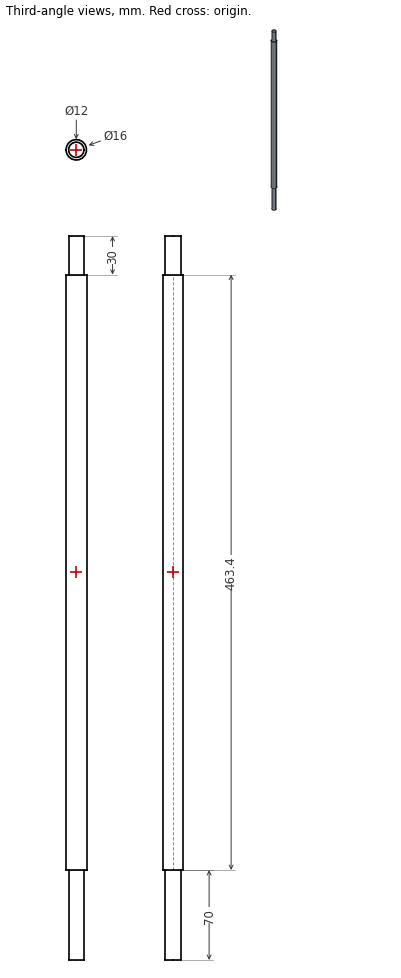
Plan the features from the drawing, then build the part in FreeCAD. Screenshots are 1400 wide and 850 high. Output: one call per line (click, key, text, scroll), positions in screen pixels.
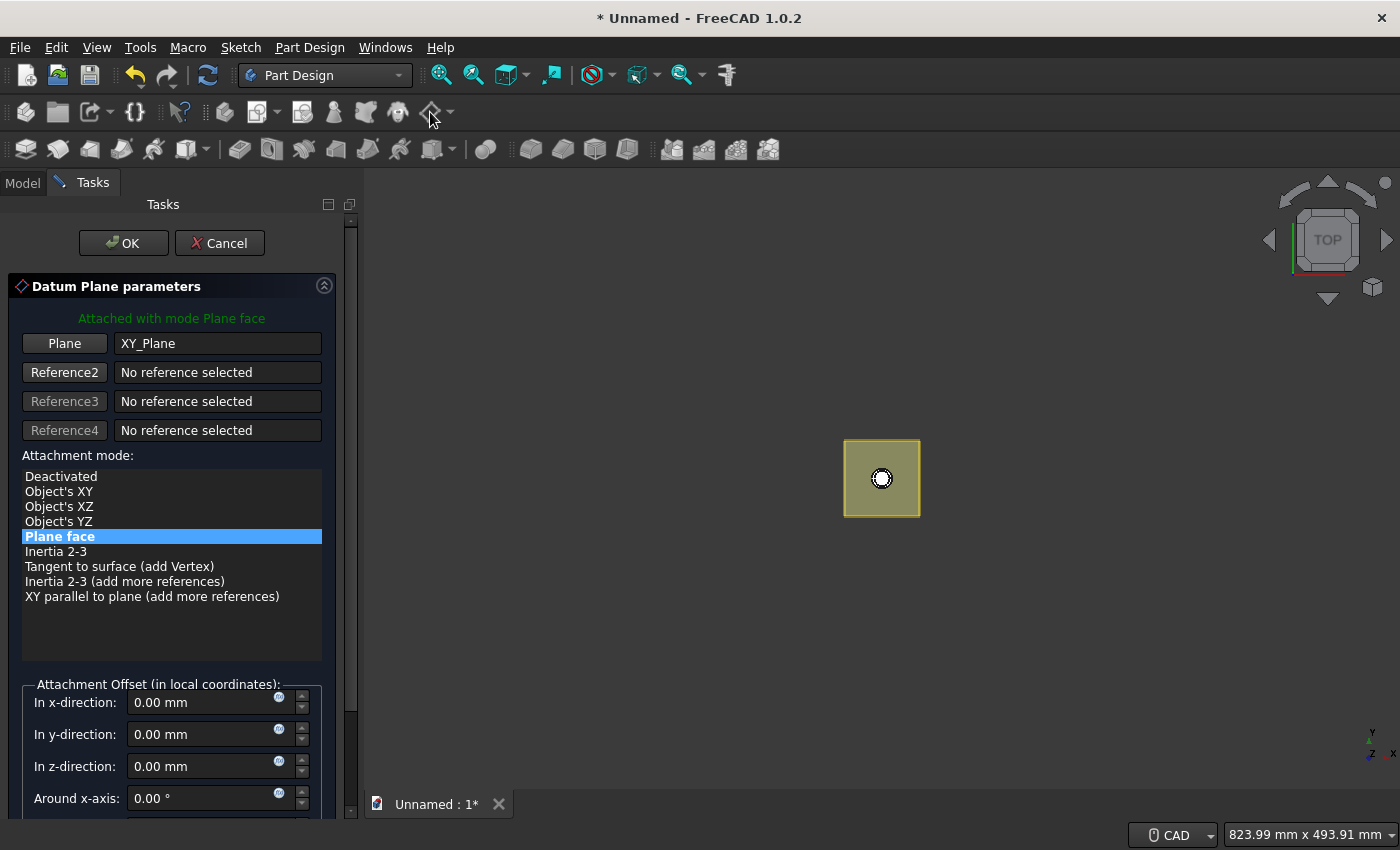
triple_click(210, 766)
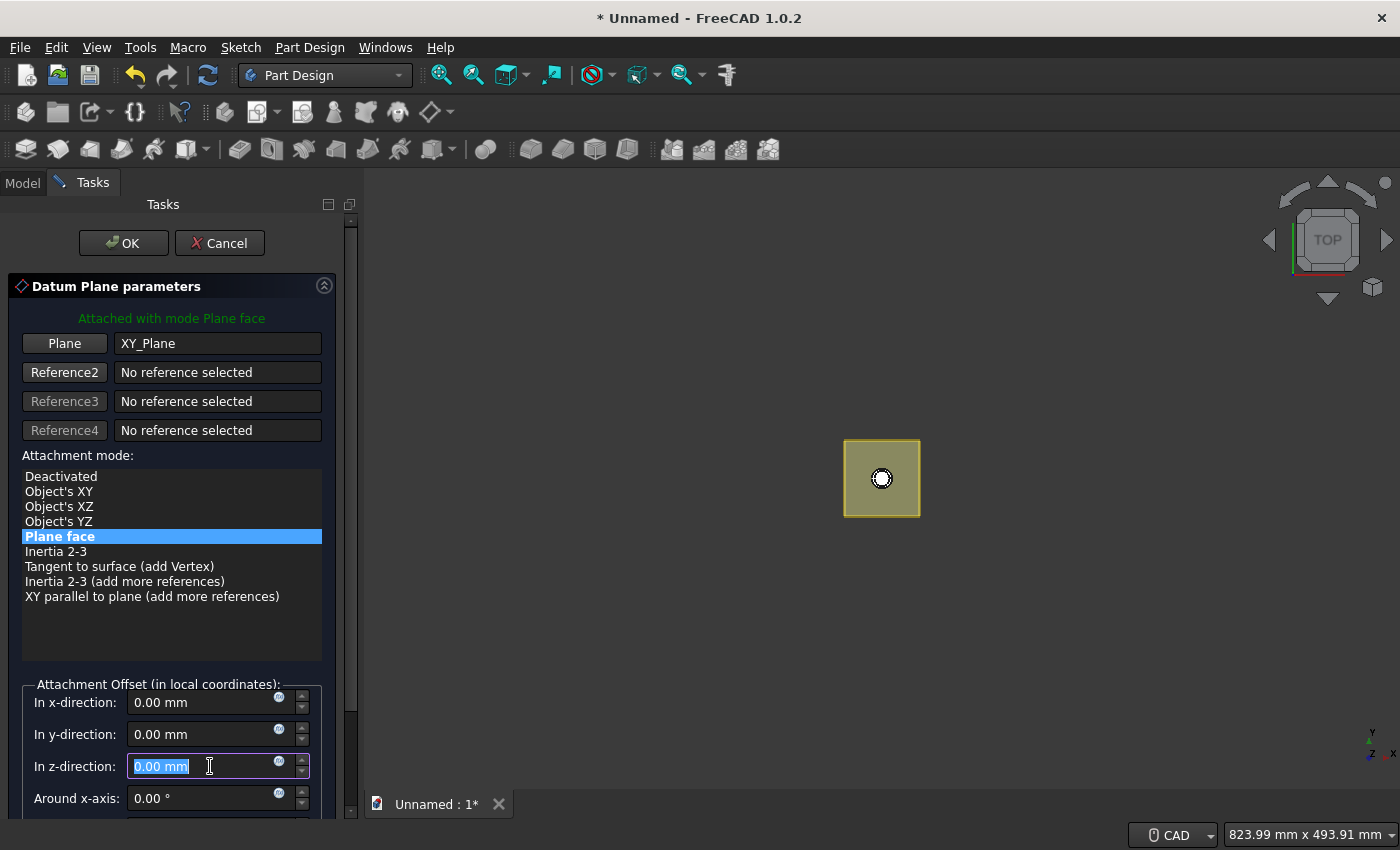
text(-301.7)
key(Tab)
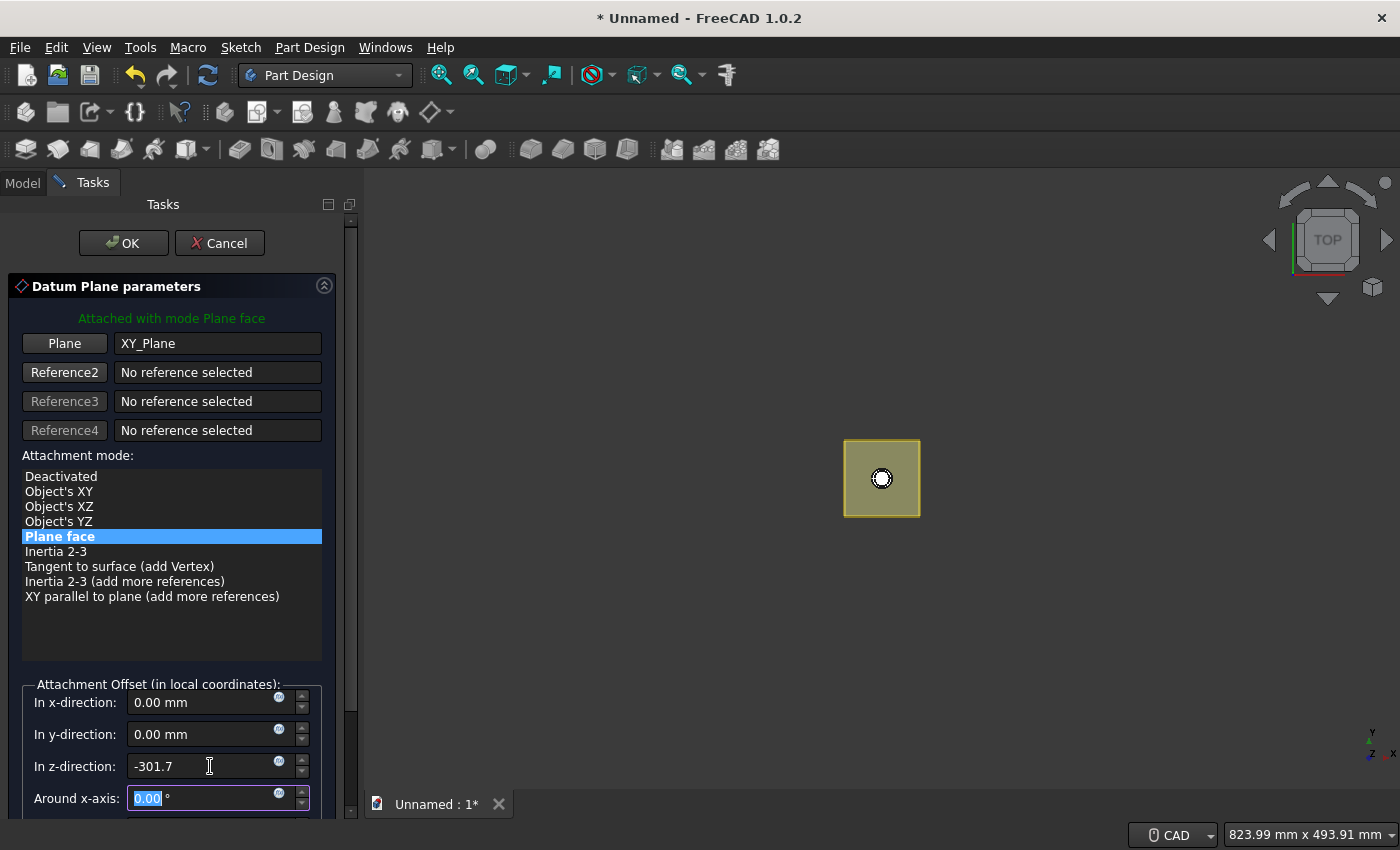
click(124, 243)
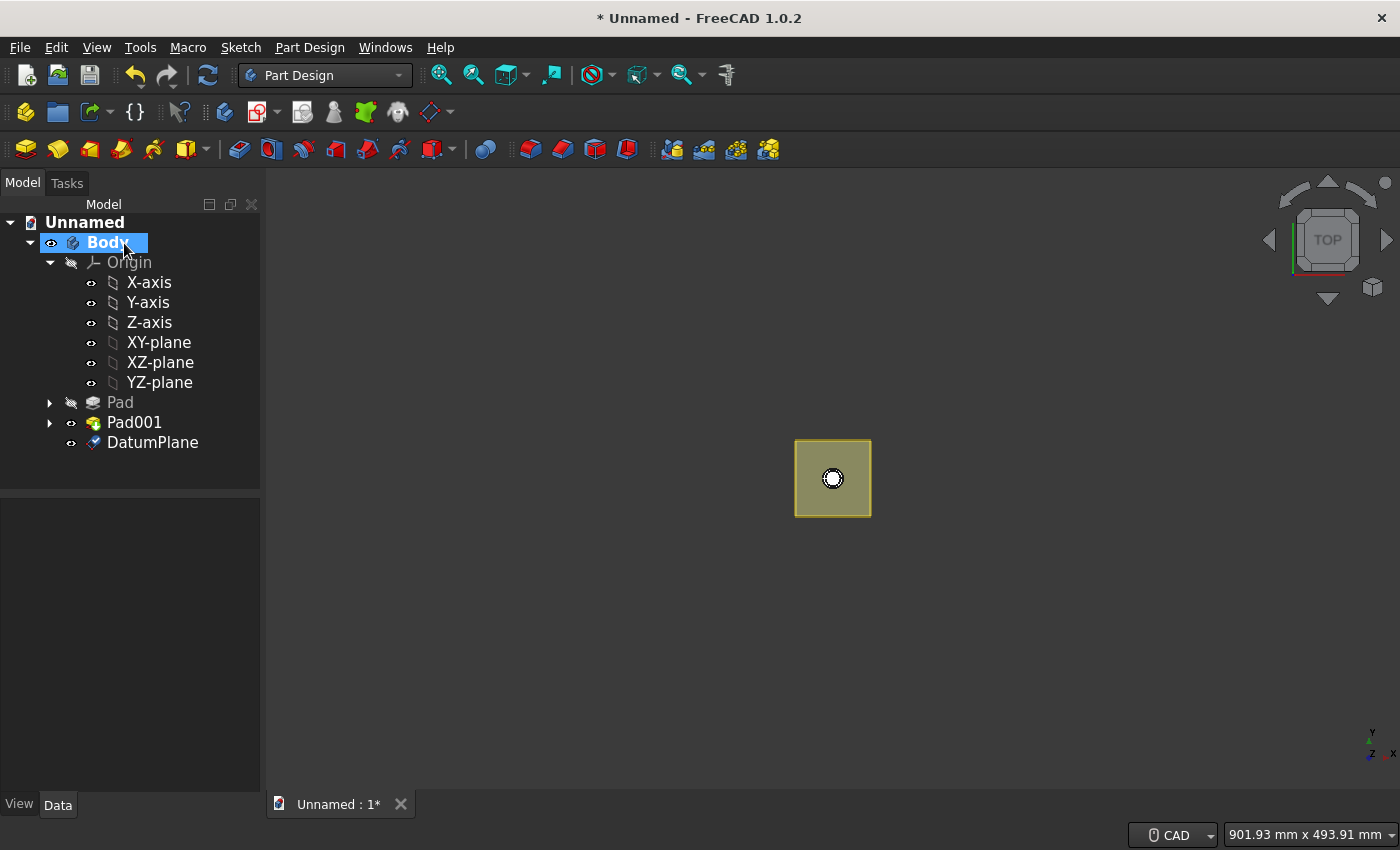
click(116, 443)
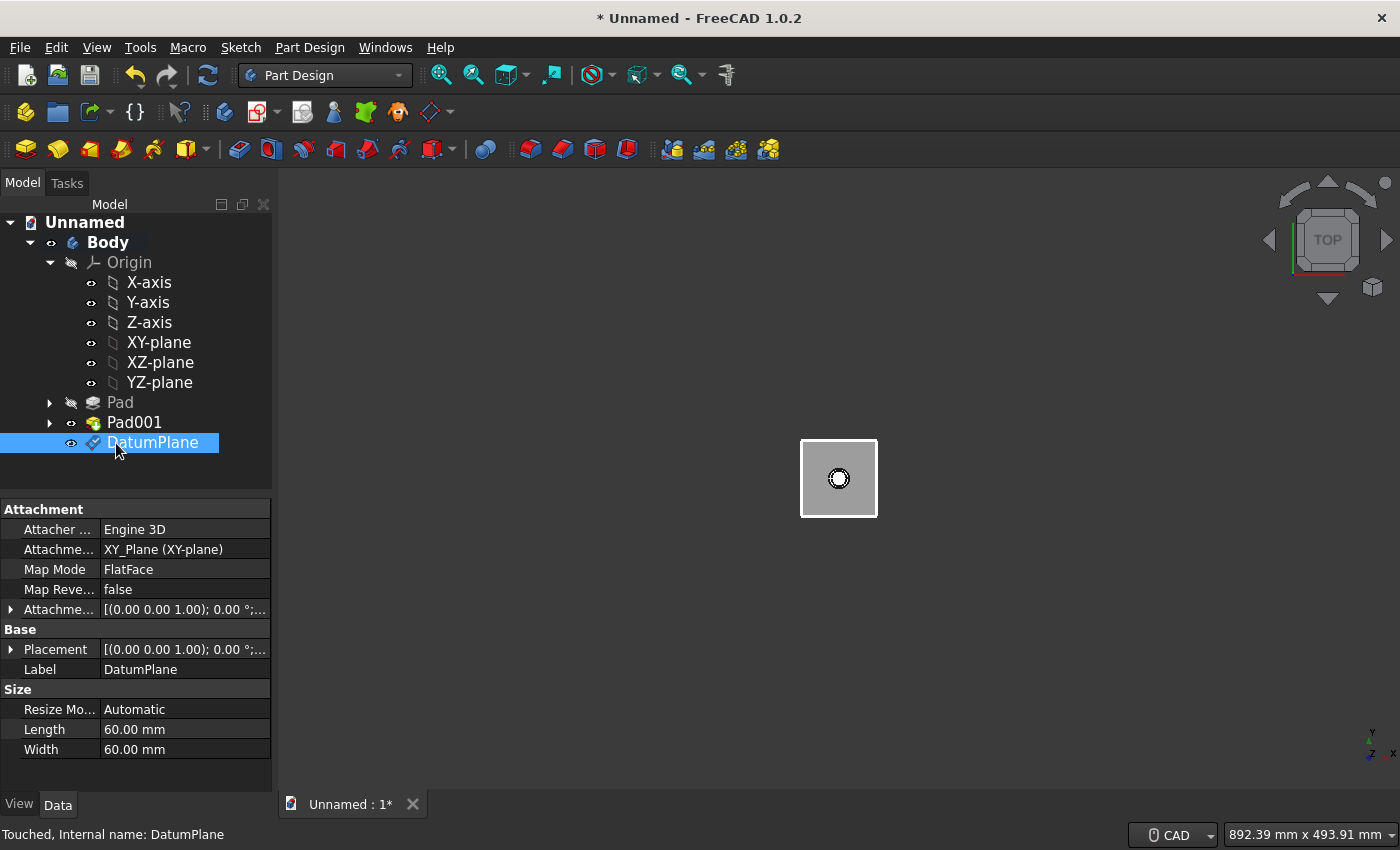
click(258, 112)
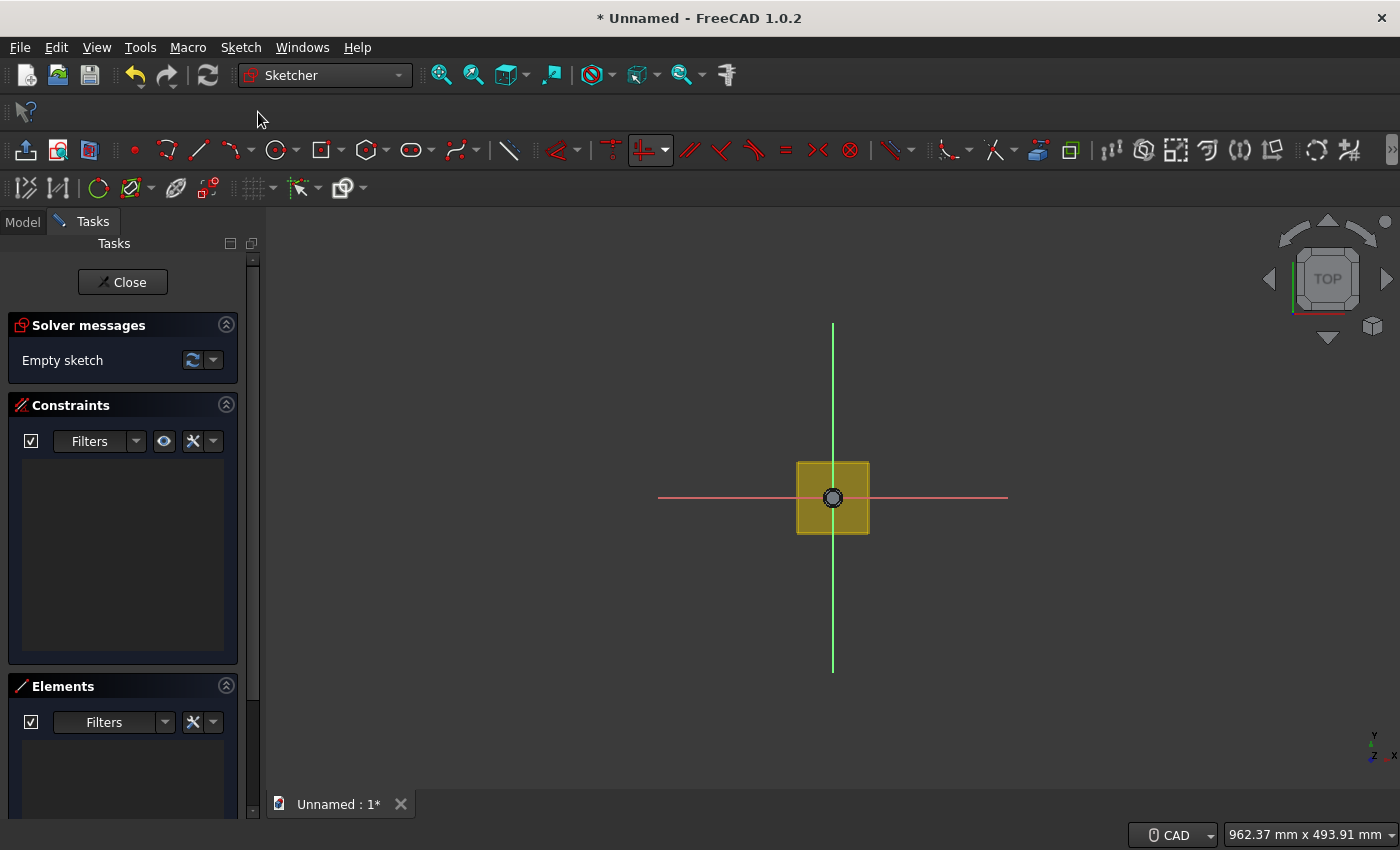
click(90, 150)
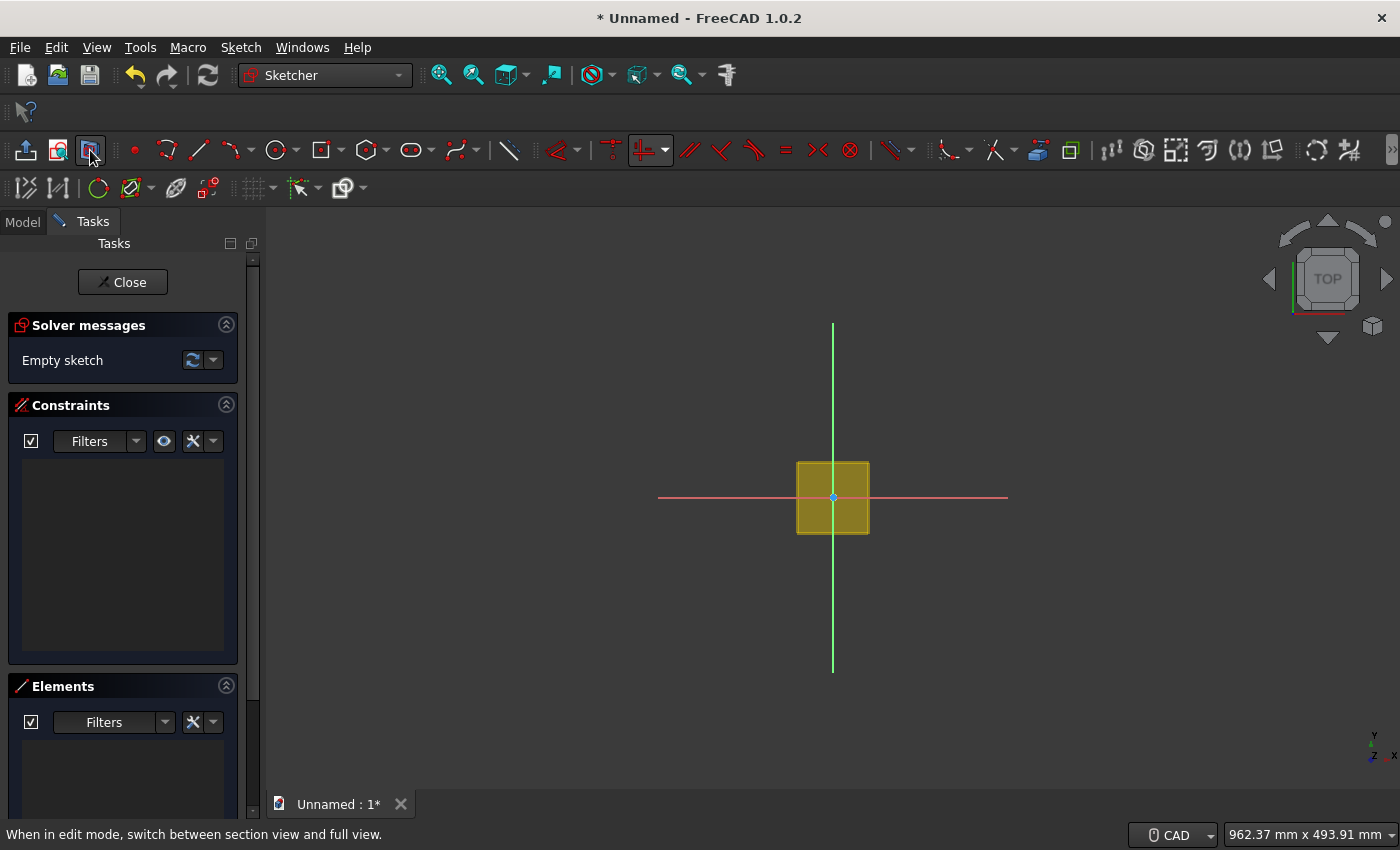
scroll(837, 498, up, 15)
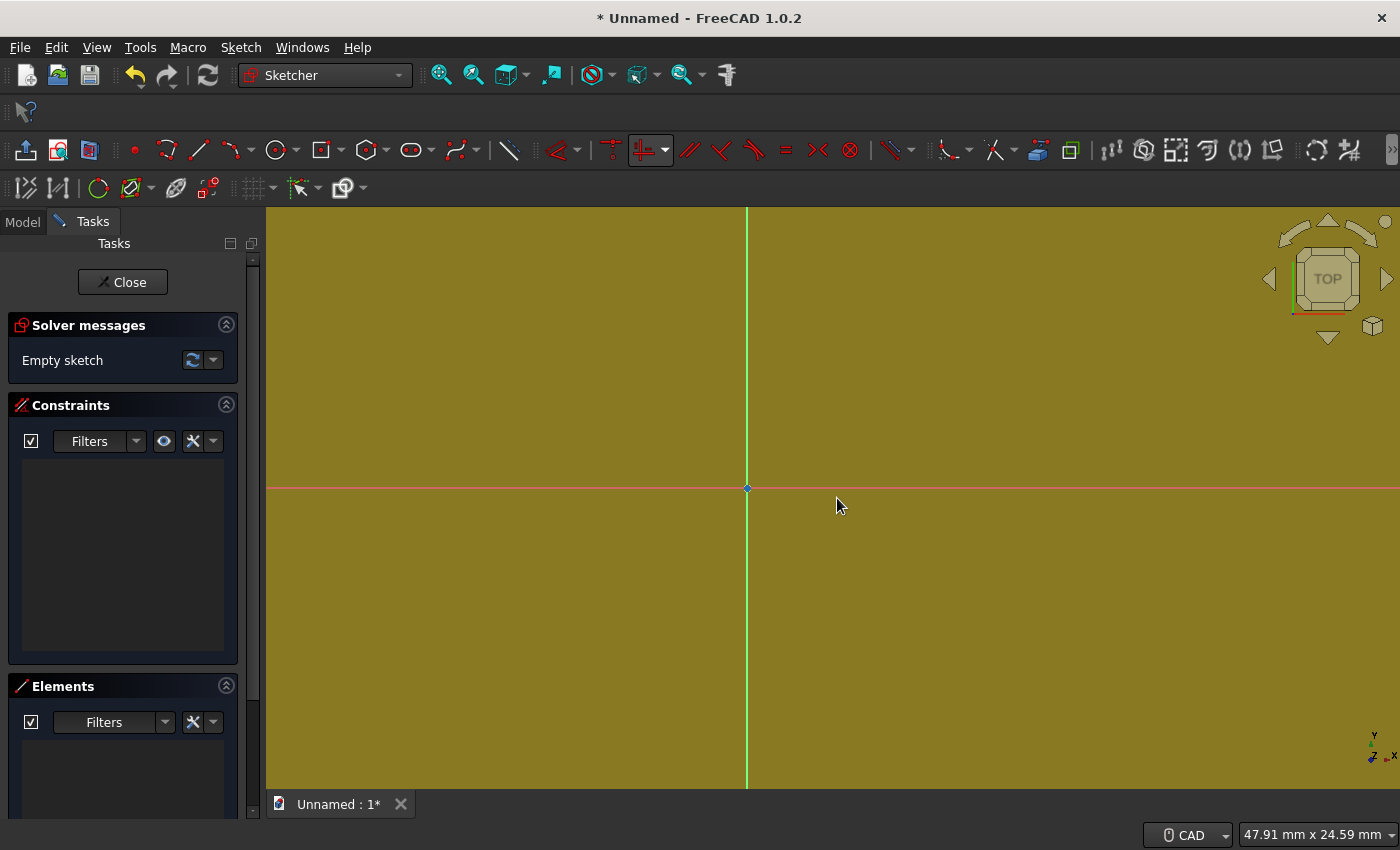
click(276, 150)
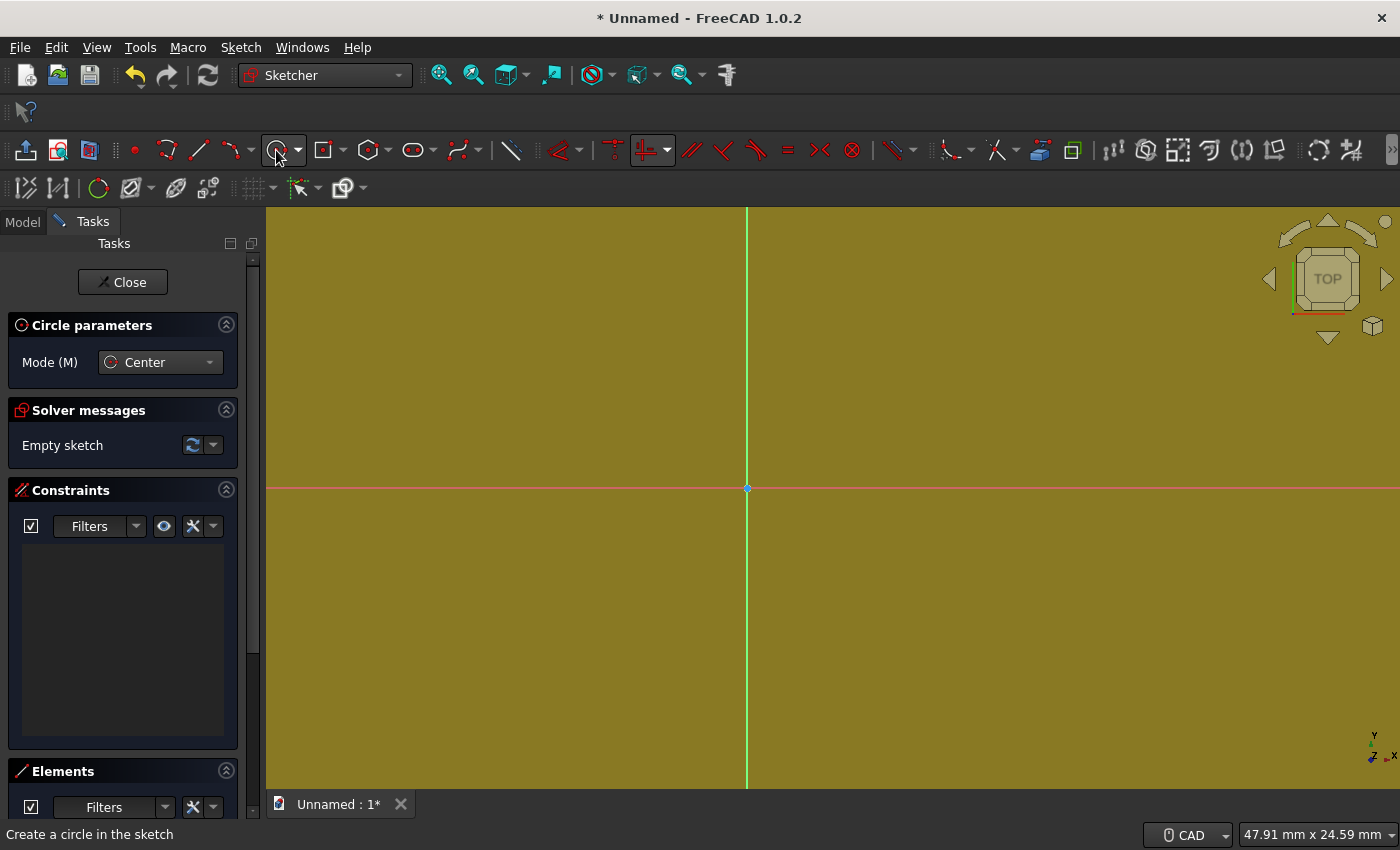
click(747, 488)
click(847, 388)
key(Escape)